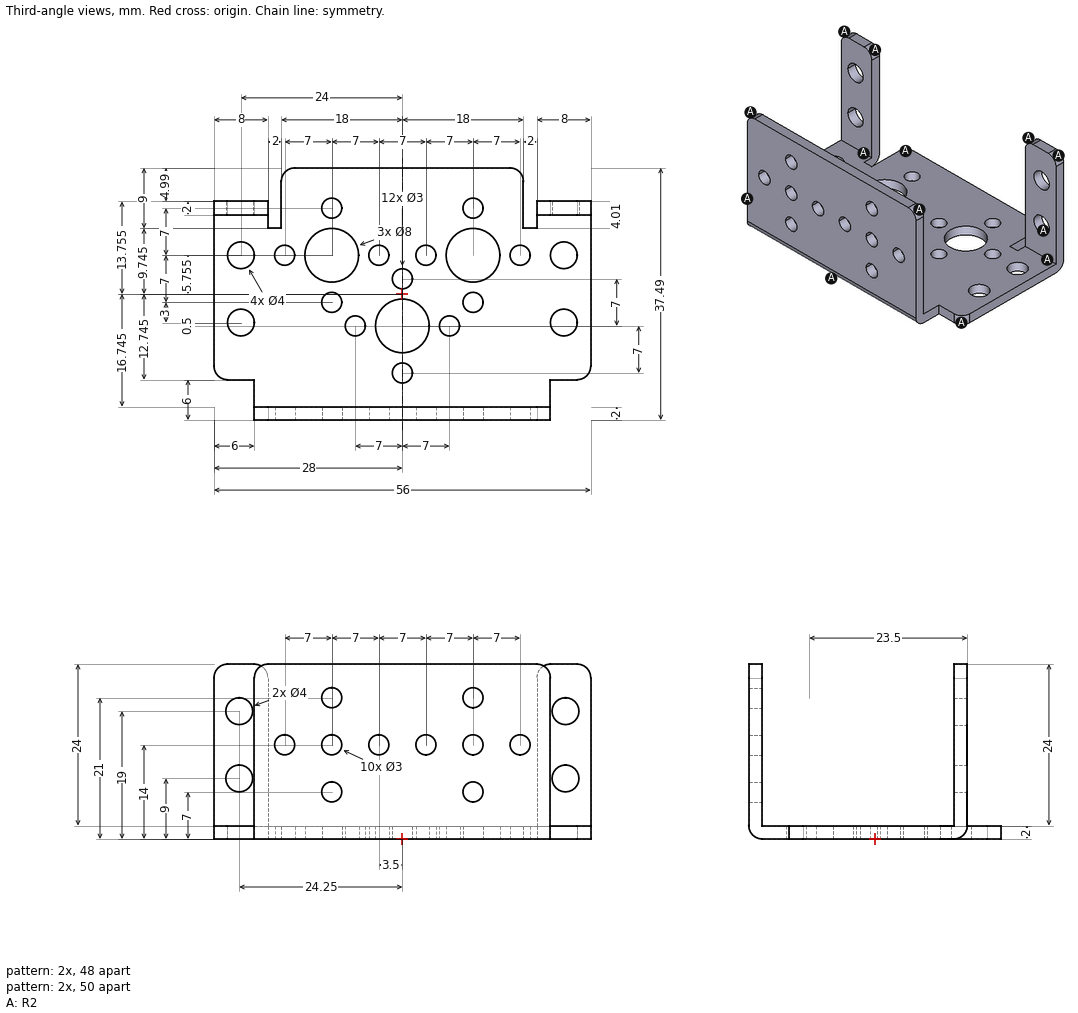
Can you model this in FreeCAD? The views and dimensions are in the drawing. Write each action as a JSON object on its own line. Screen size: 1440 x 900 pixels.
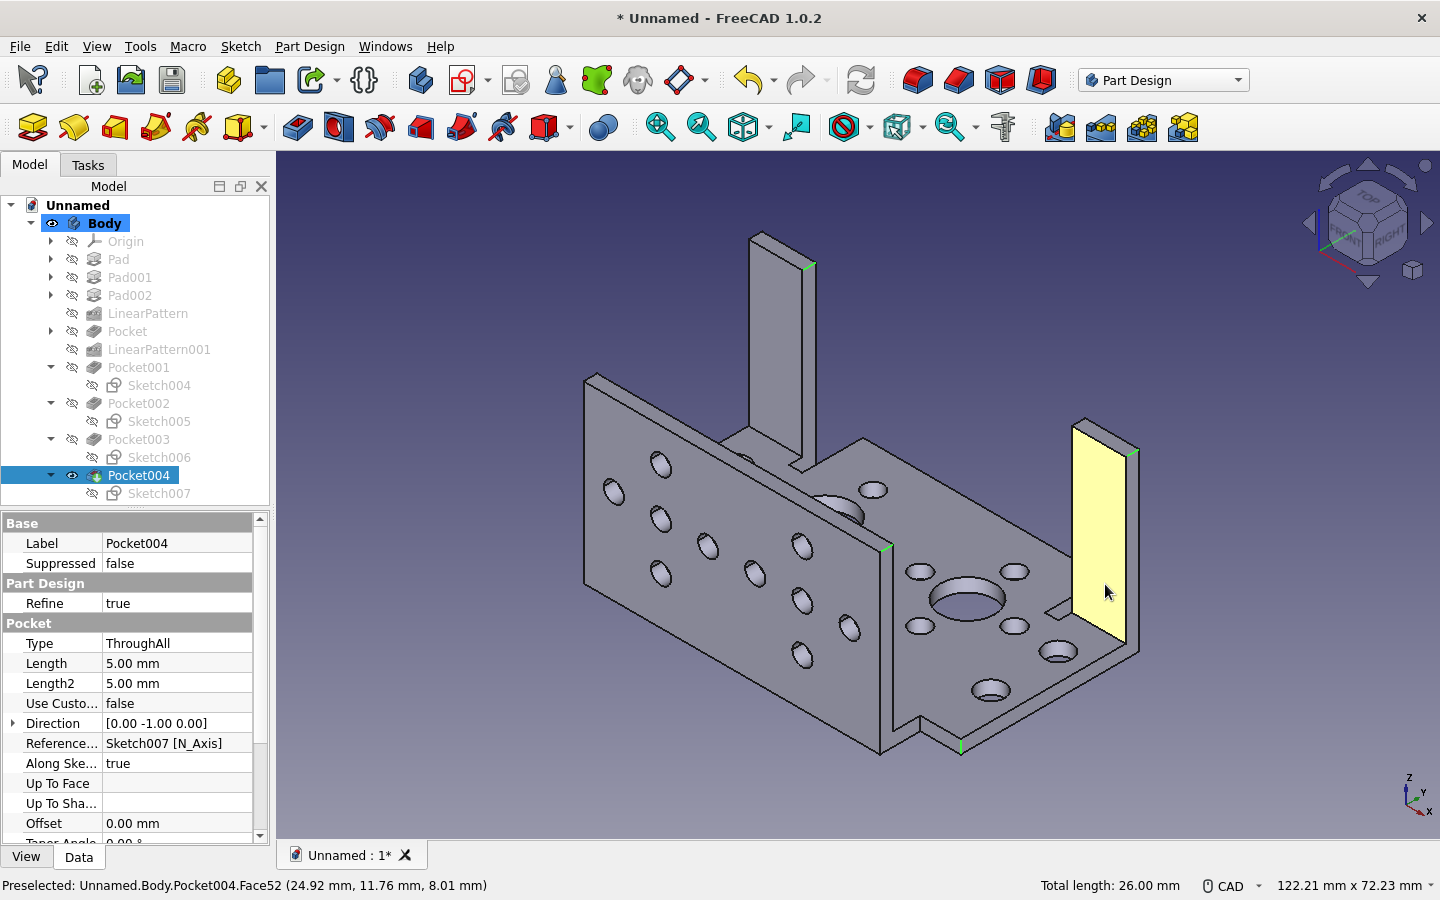
{"action": "key", "text": "2"}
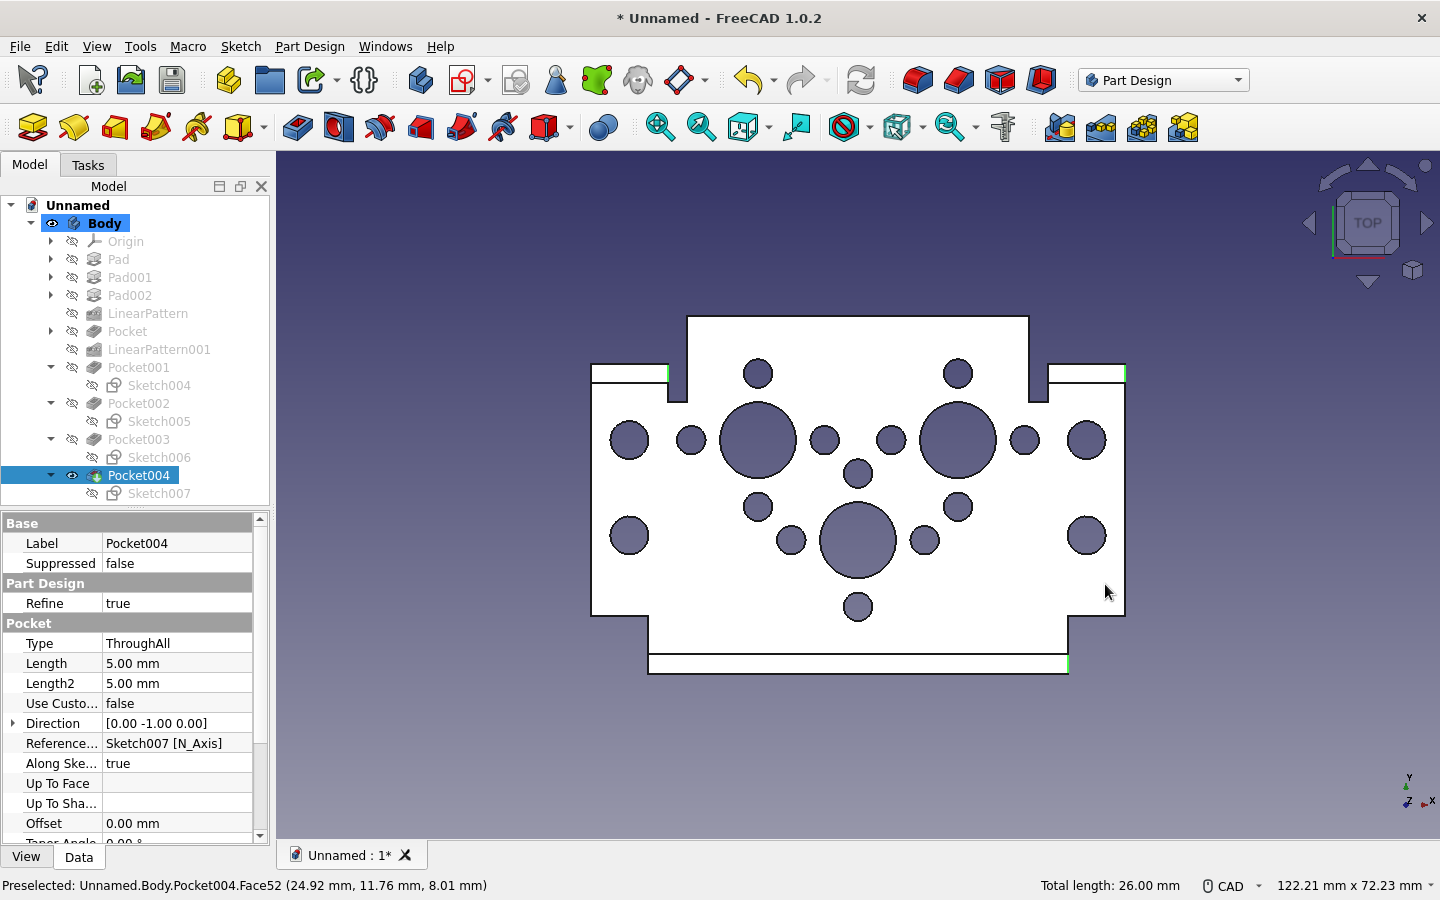
{"action": "left_click", "coordinate": [591, 373], "text": "ctrl"}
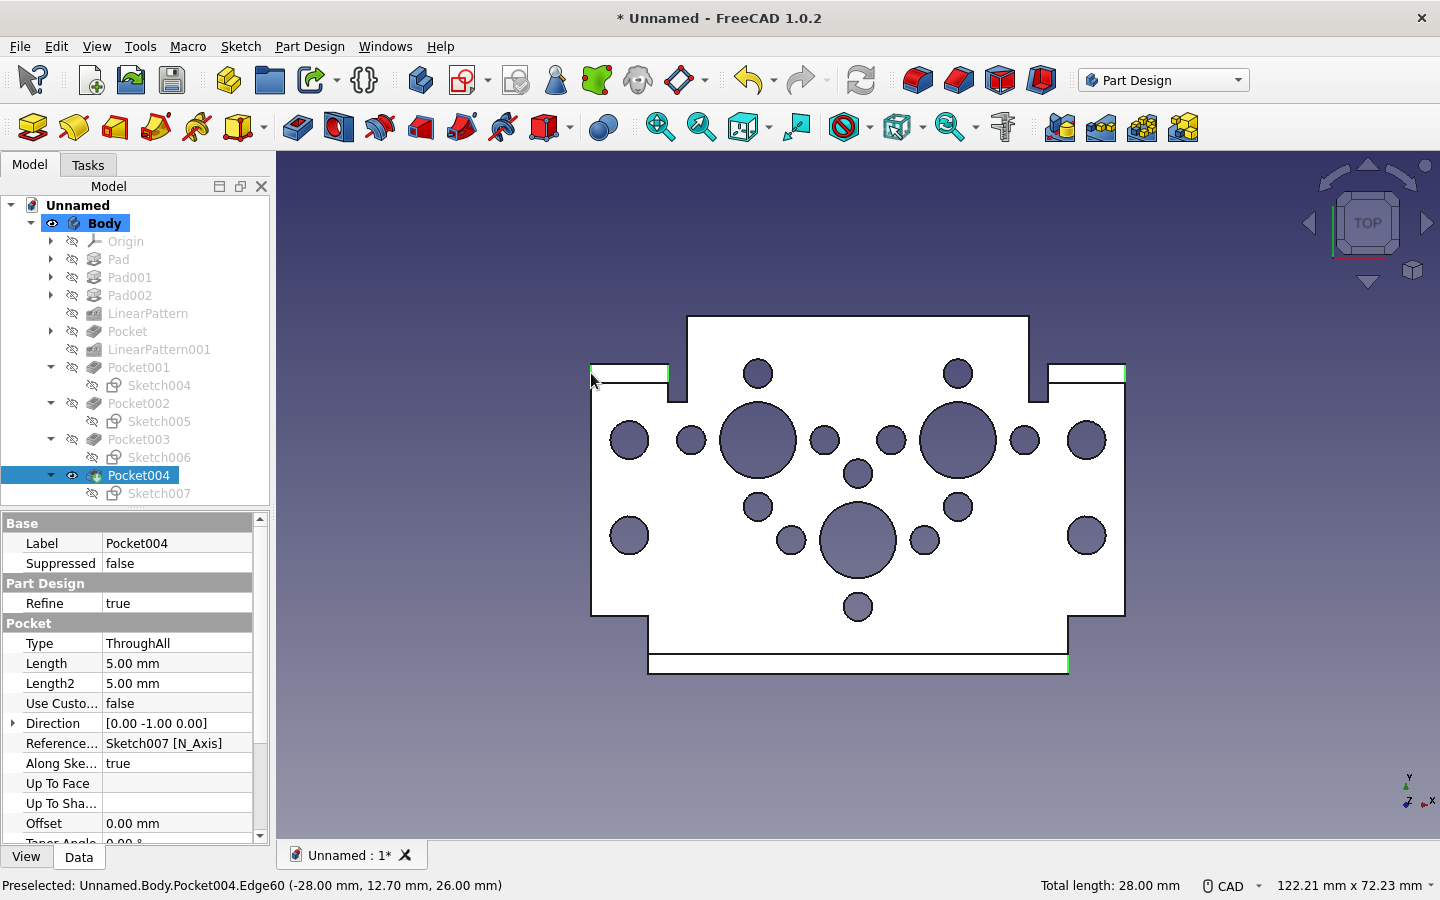
{"action": "left_click", "coordinate": [1048, 373], "text": "ctrl"}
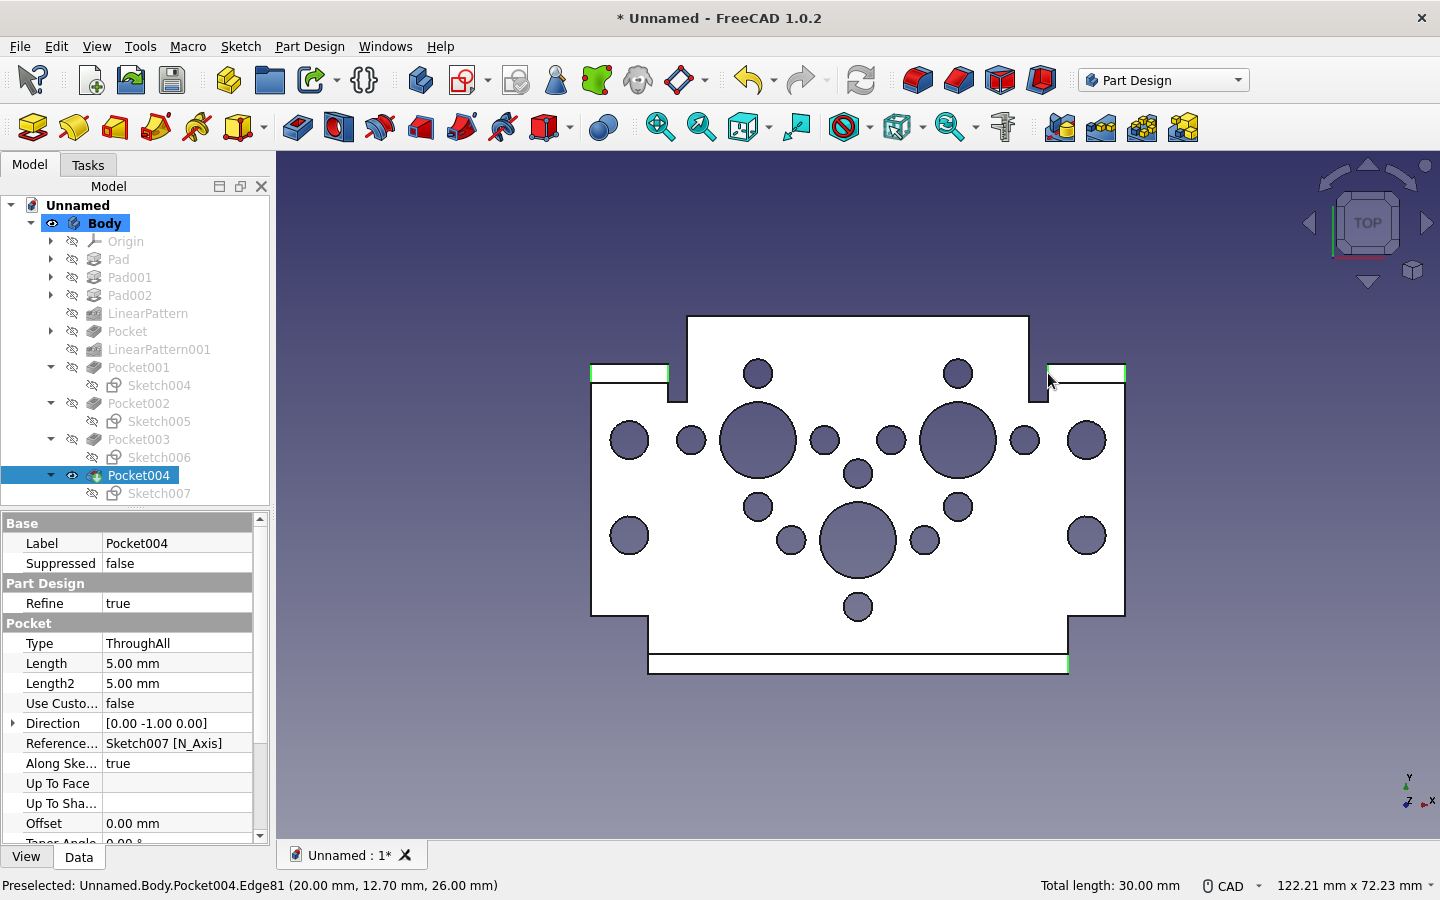
{"action": "left_click", "coordinate": [648, 663], "text": "ctrl"}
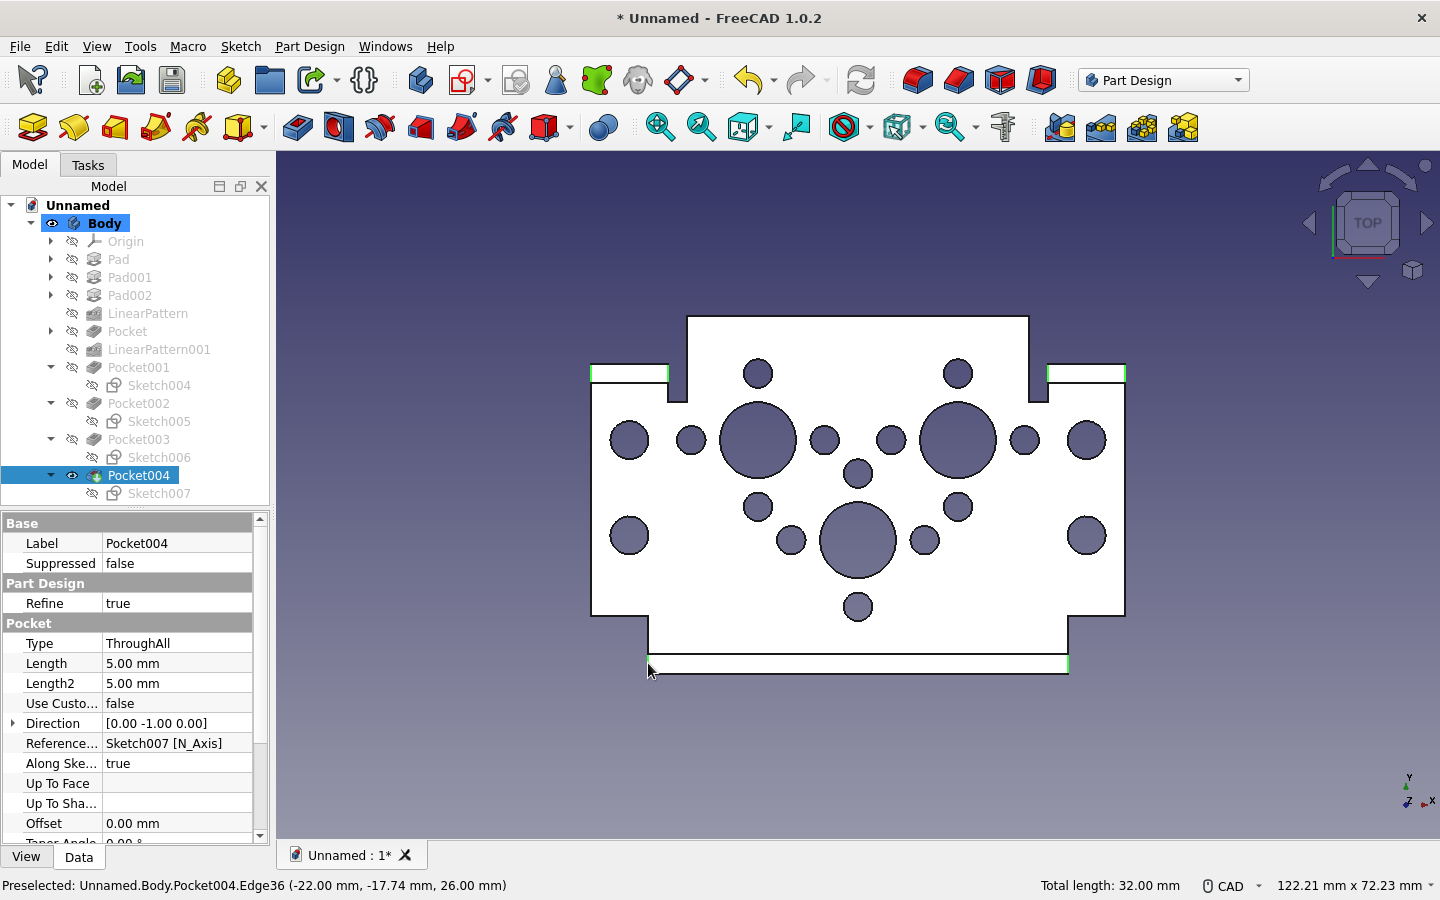
{"action": "scroll", "coordinate": [1029, 315], "scroll_direction": "up", "scroll_amount": 4}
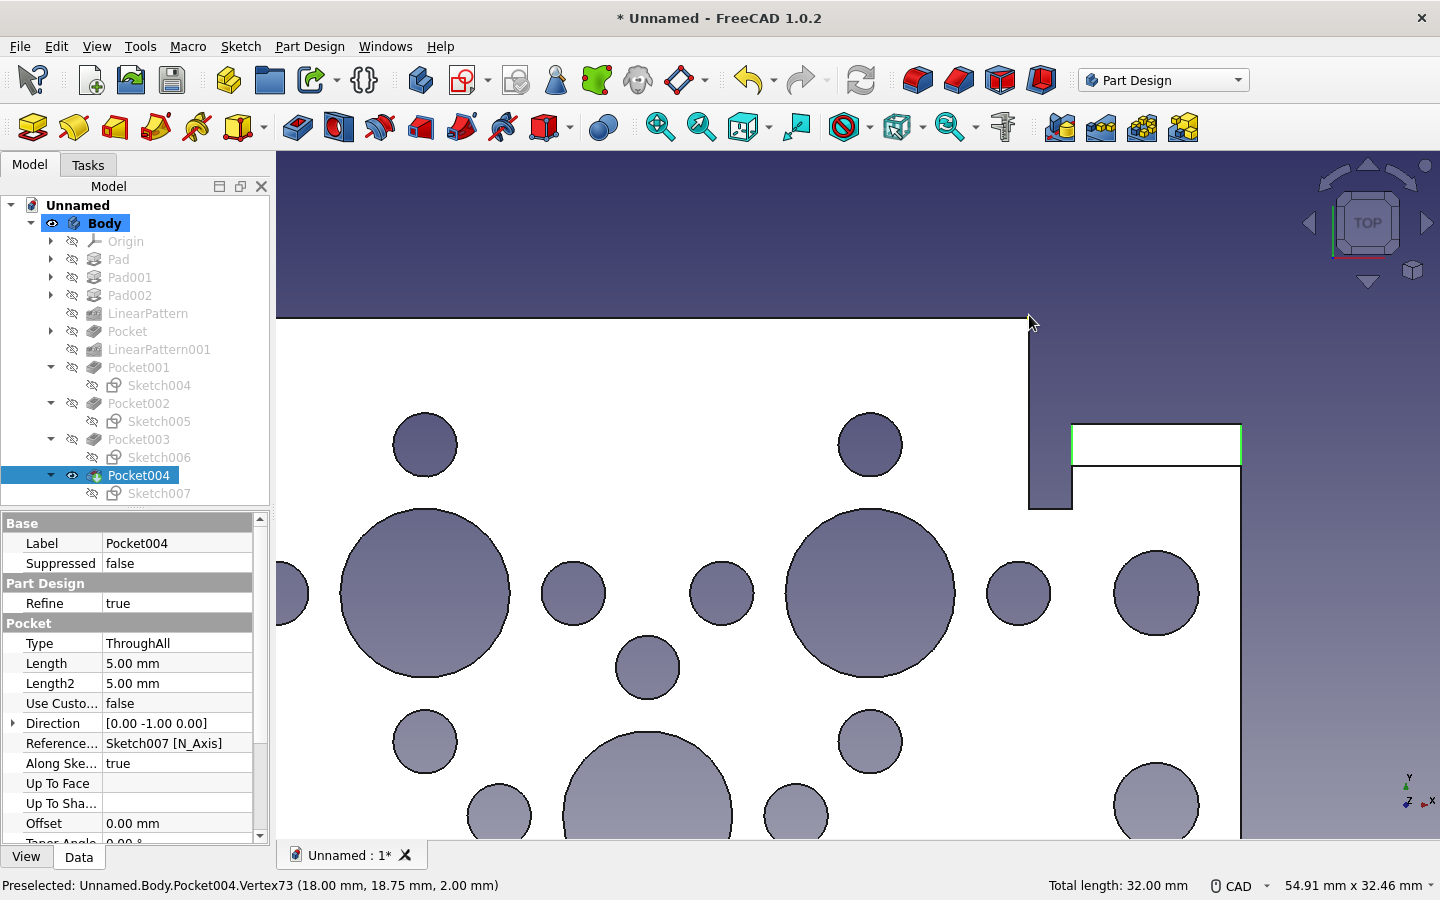
{"action": "key", "text": "v f"}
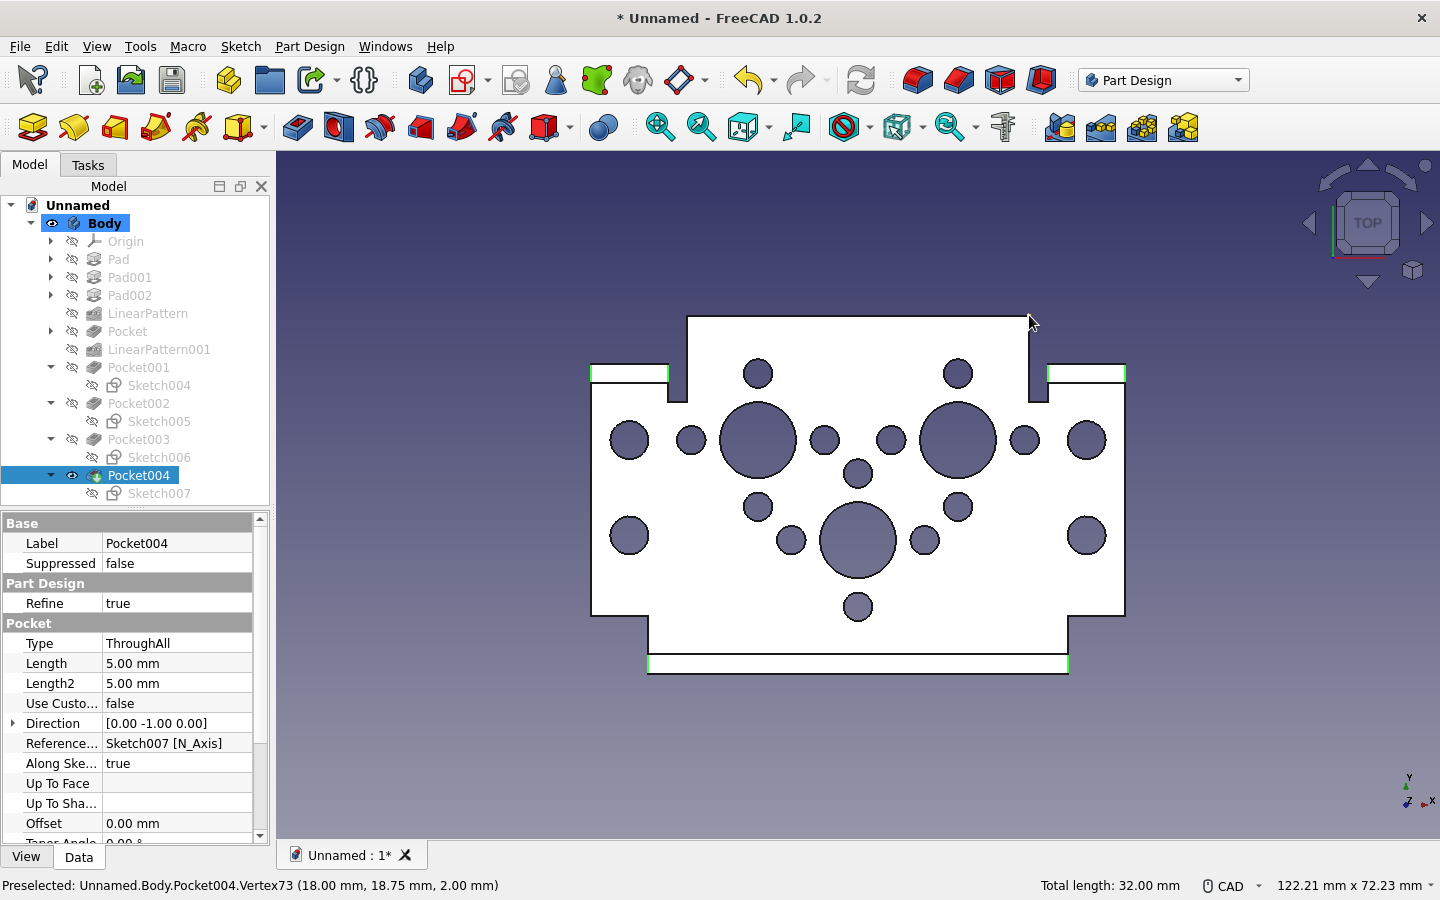
{"action": "key", "text": "1"}